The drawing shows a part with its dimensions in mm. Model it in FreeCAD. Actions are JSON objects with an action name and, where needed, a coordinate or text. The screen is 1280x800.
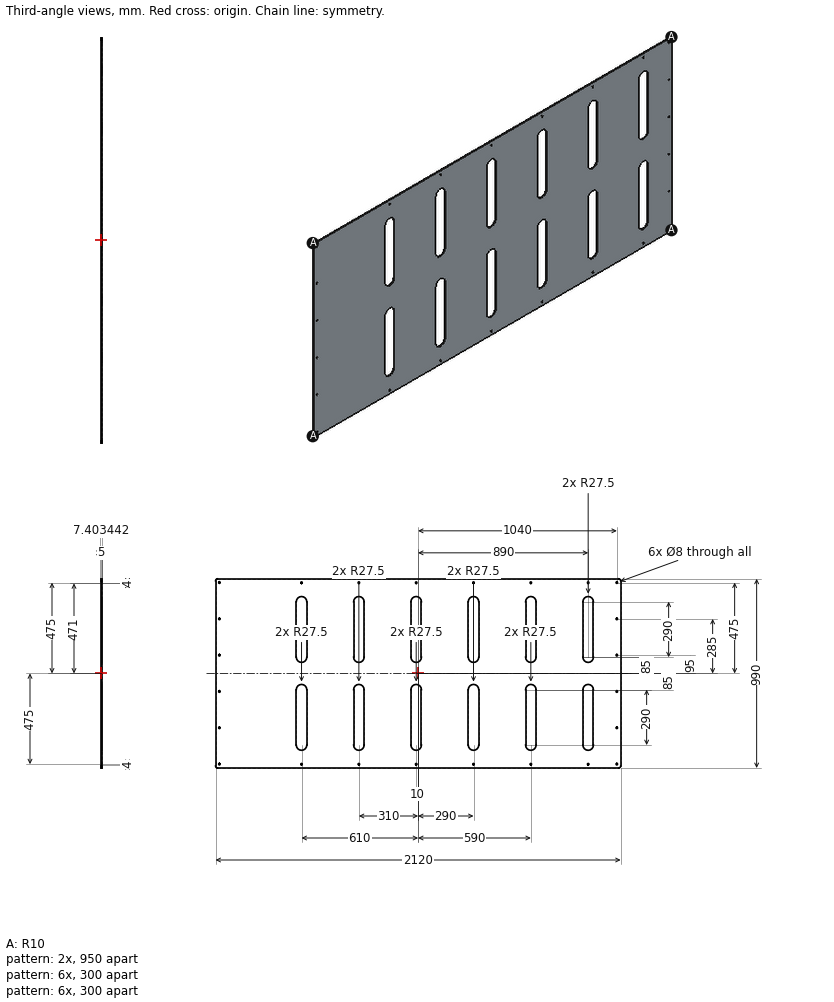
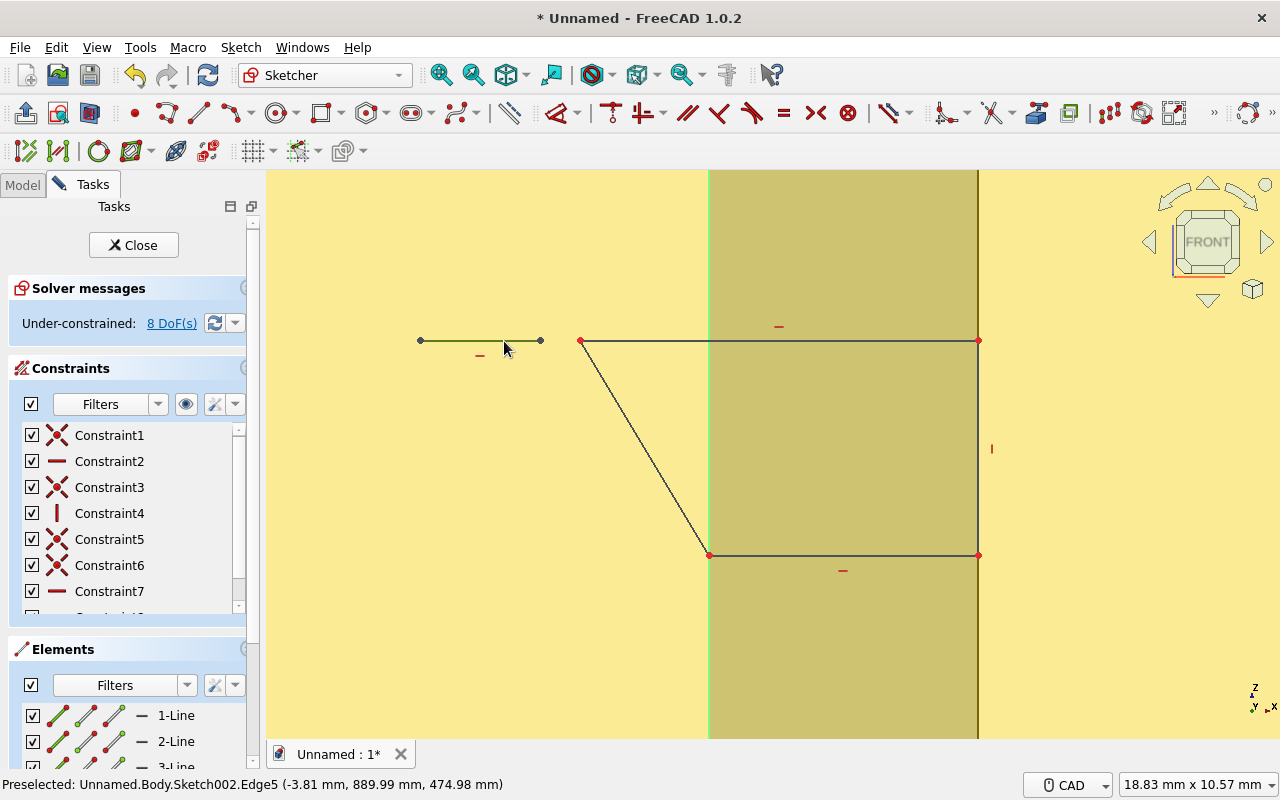
{"action": "left_click", "coordinate": [510, 114]}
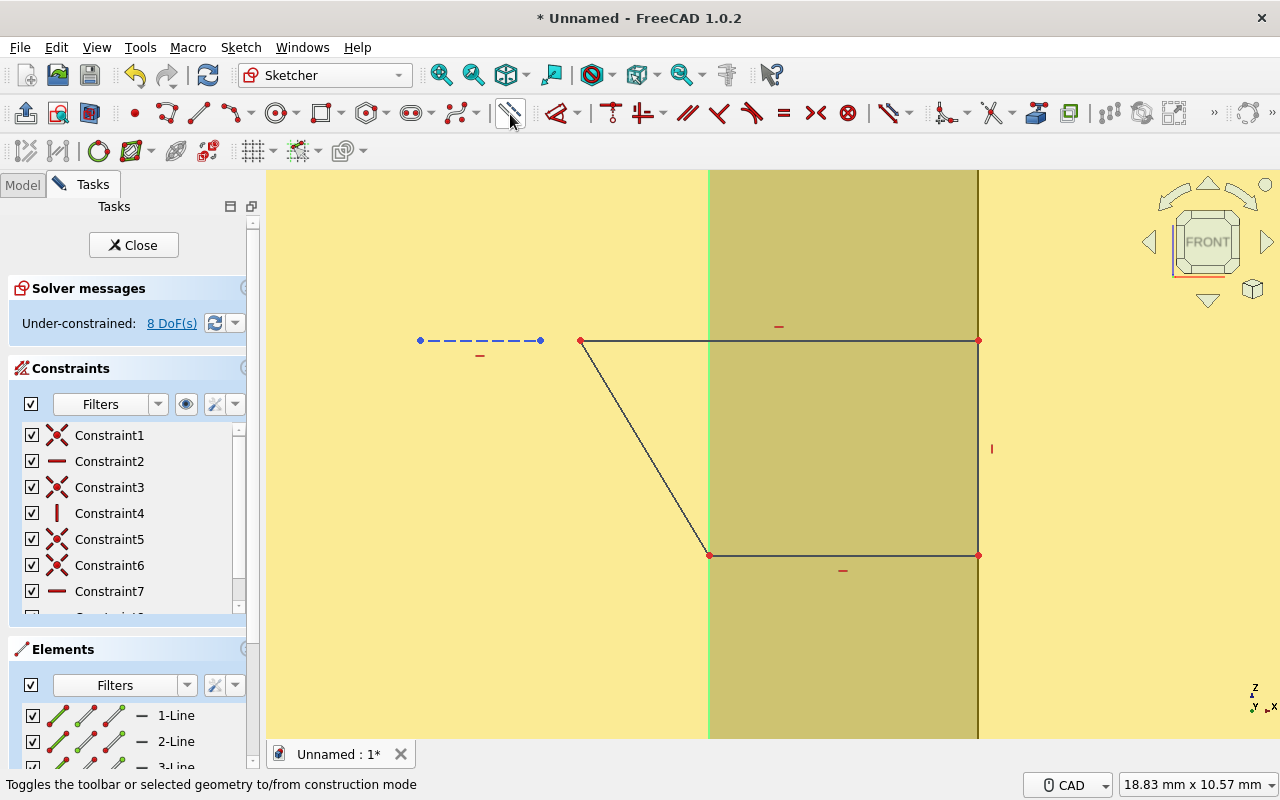
{"action": "left_click", "coordinate": [709, 556]}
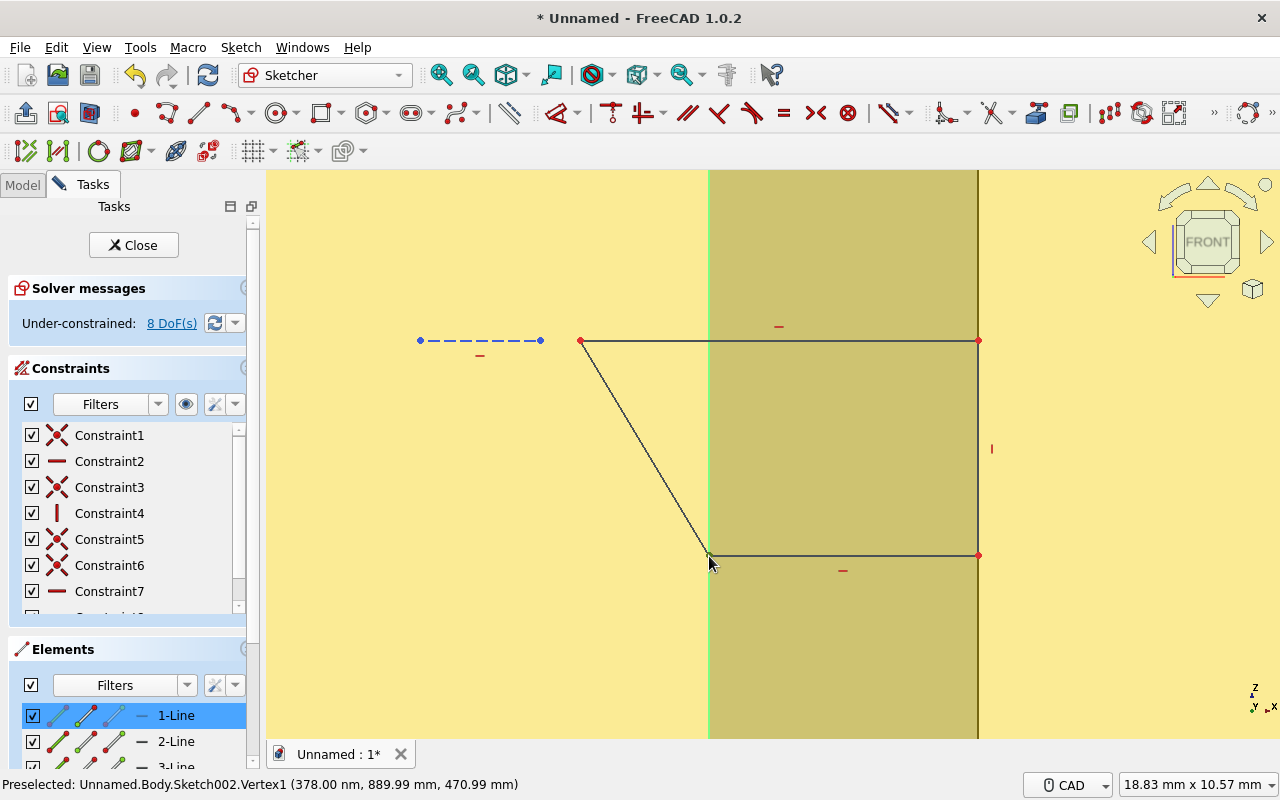
{"action": "left_click", "coordinate": [709, 674]}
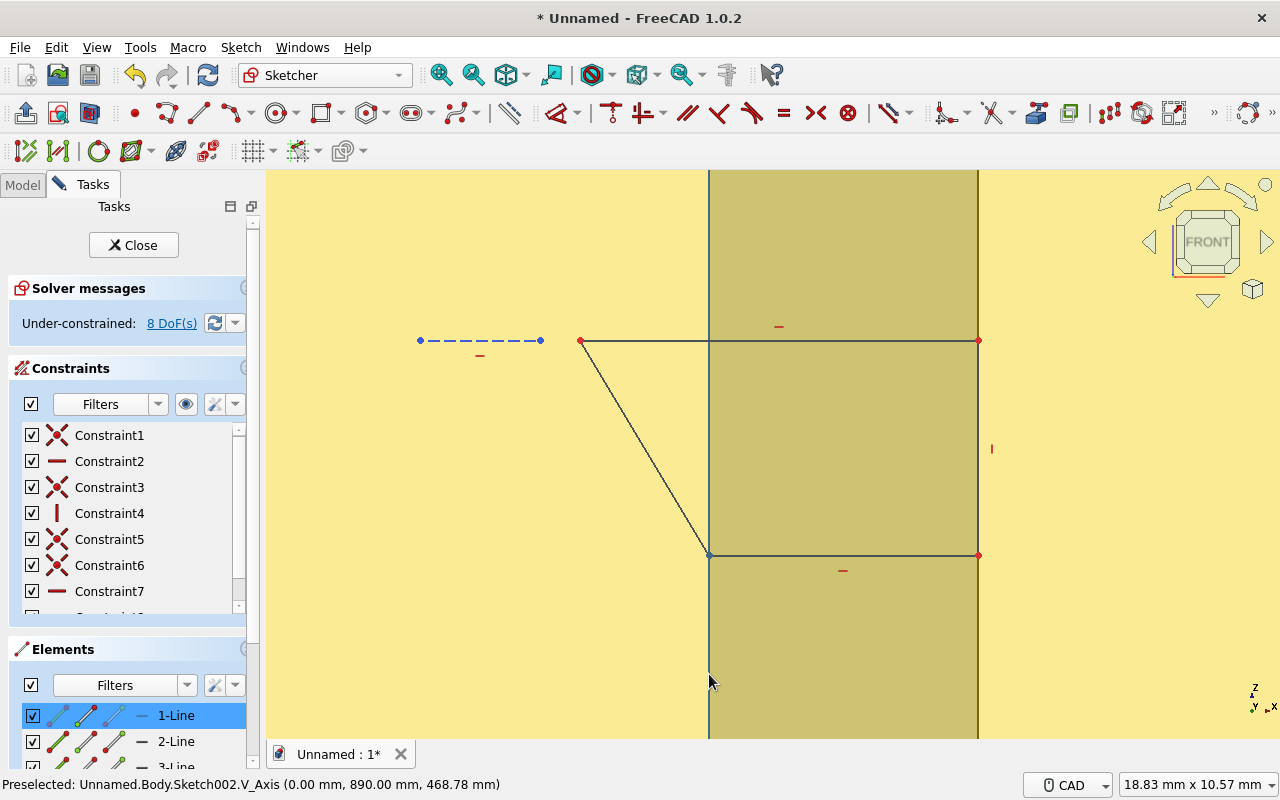
{"action": "left_click", "coordinate": [612, 114]}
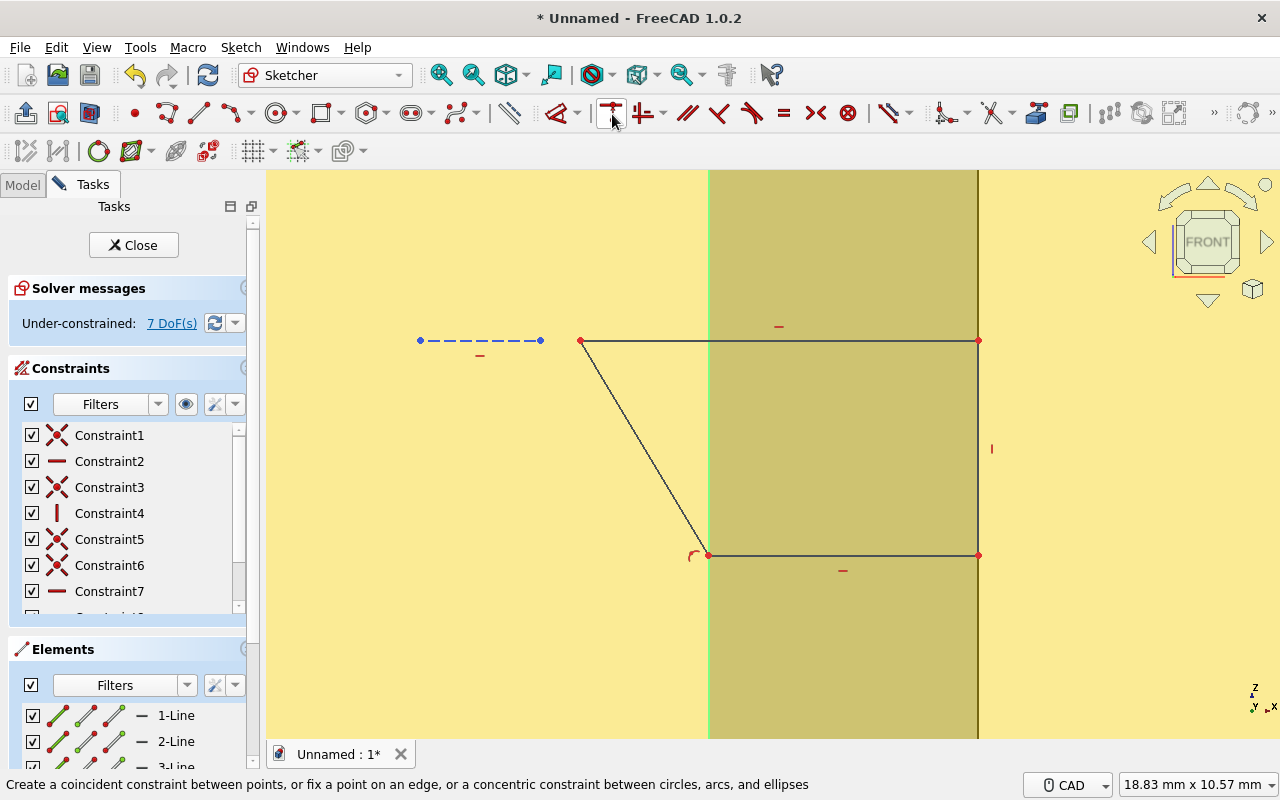
{"action": "key", "text": "d"}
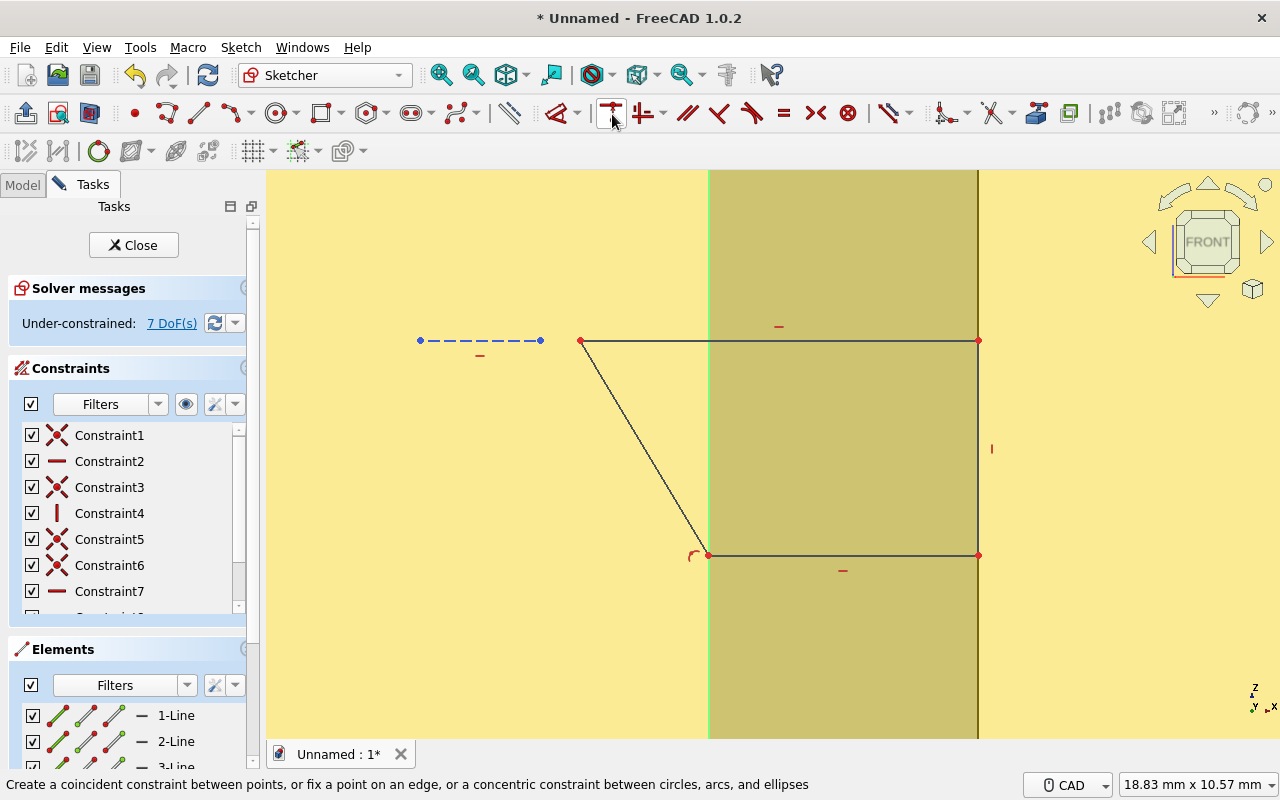
{"action": "left_click", "coordinate": [978, 406]}
{"action": "left_click", "coordinate": [1012, 448]}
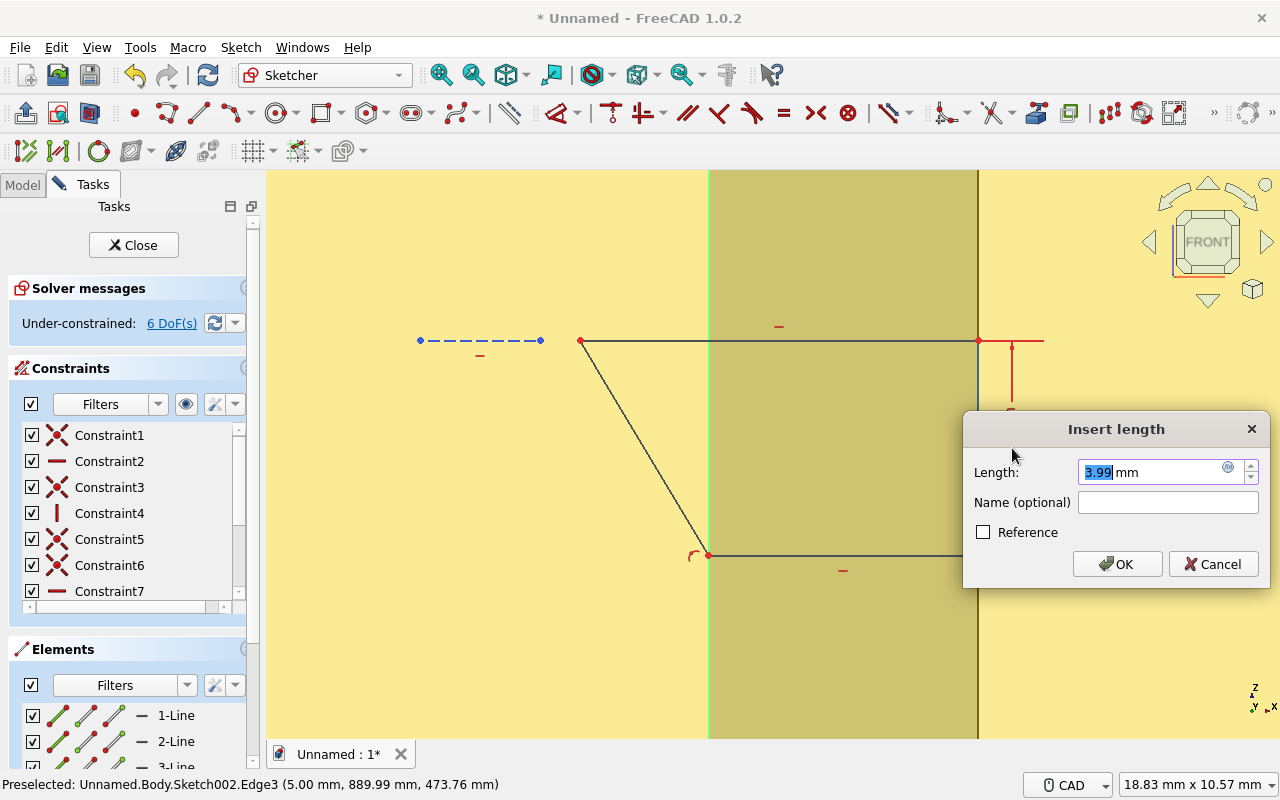
{"action": "type", "text": "4"}
{"action": "key", "text": "Return"}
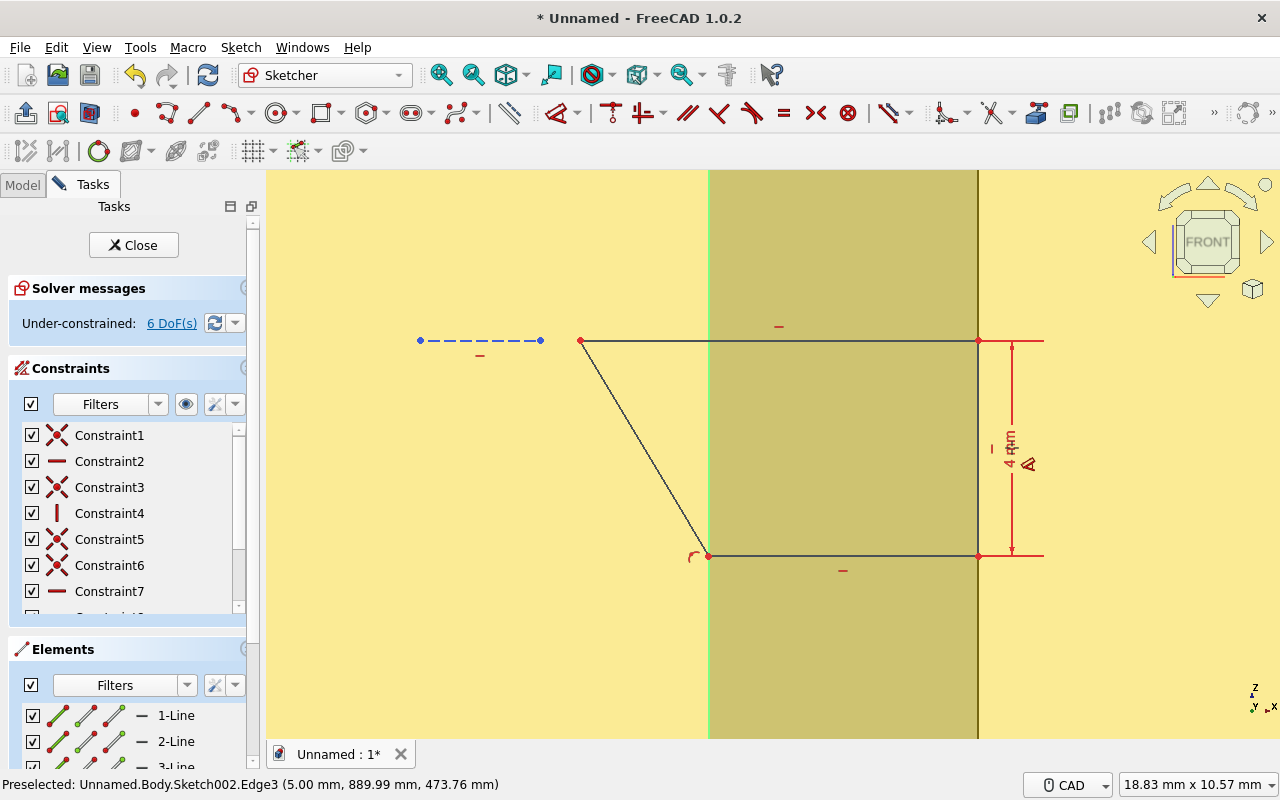
{"action": "left_click", "coordinate": [897, 556]}
{"action": "left_click", "coordinate": [843, 590]}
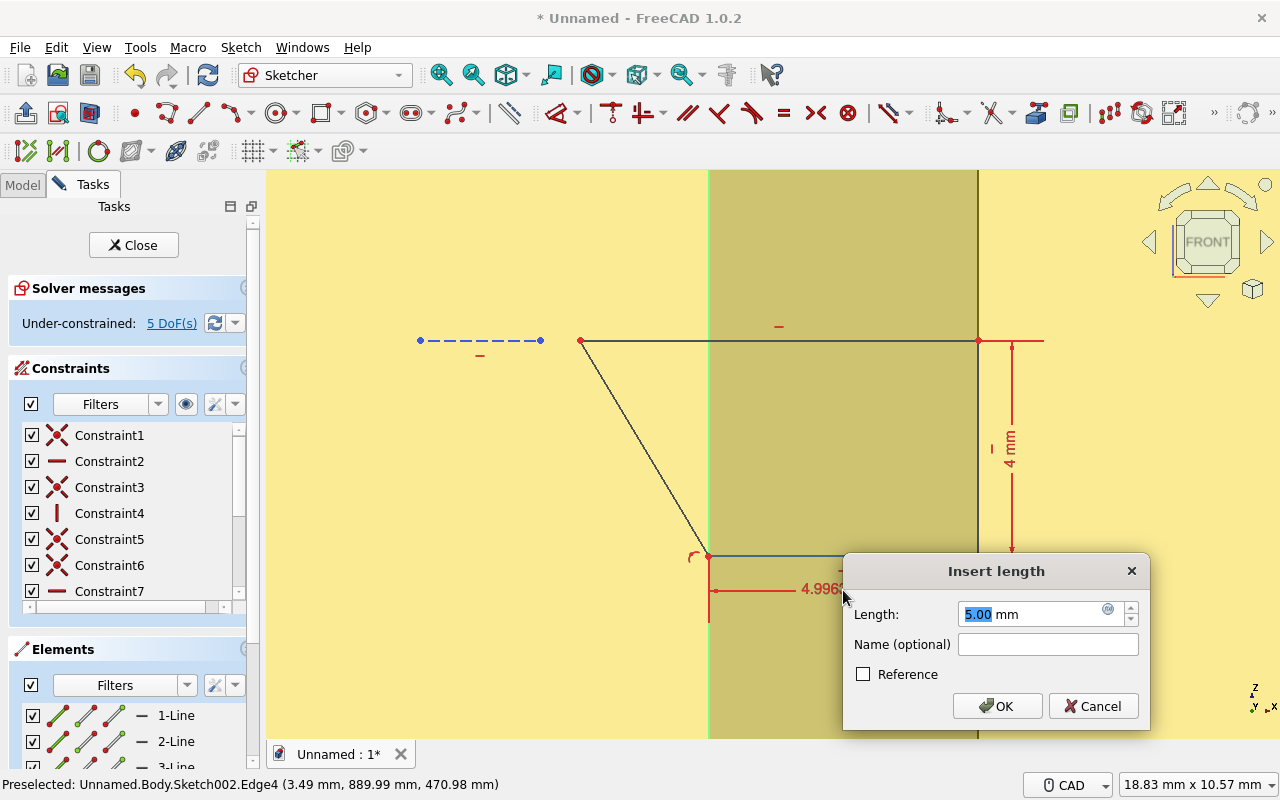
{"action": "type", "text": "5"}
{"action": "key", "text": "Return"}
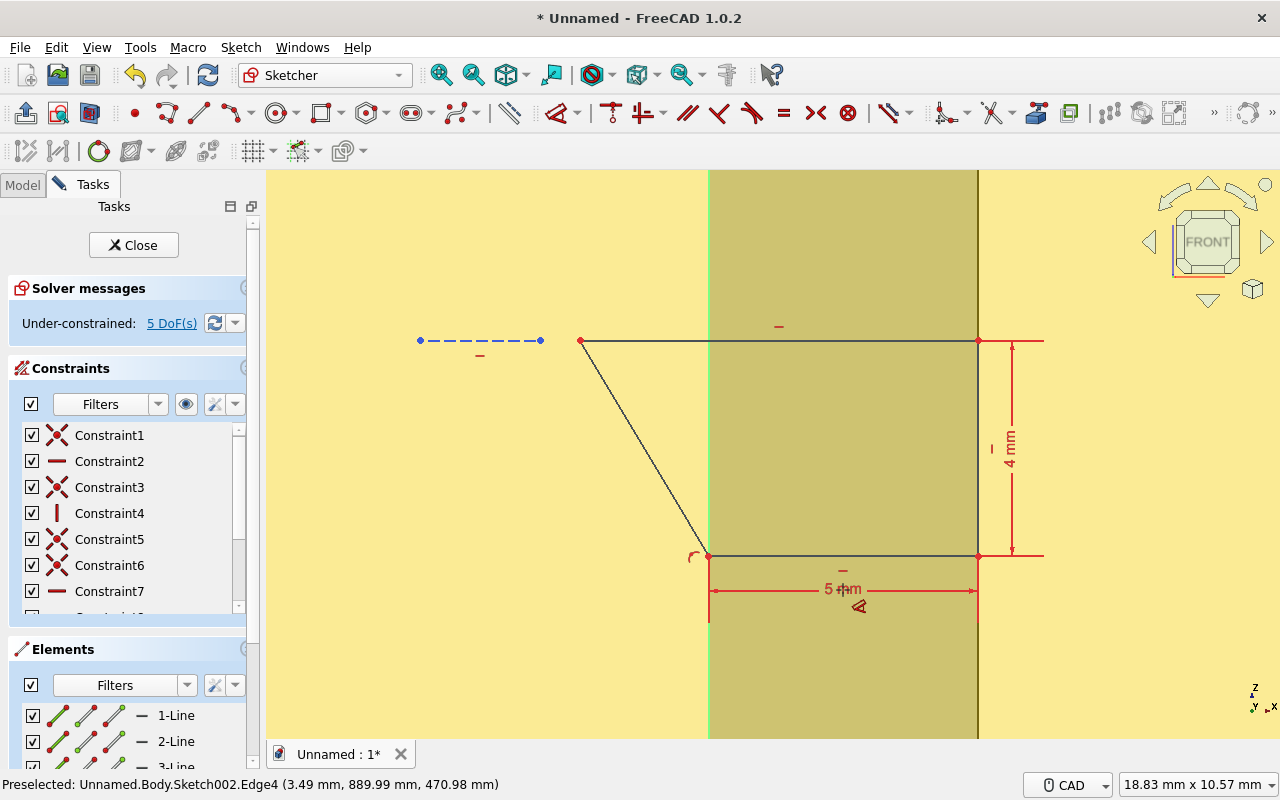
{"action": "left_click", "coordinate": [709, 556]}
{"action": "left_click", "coordinate": [743, 634]}